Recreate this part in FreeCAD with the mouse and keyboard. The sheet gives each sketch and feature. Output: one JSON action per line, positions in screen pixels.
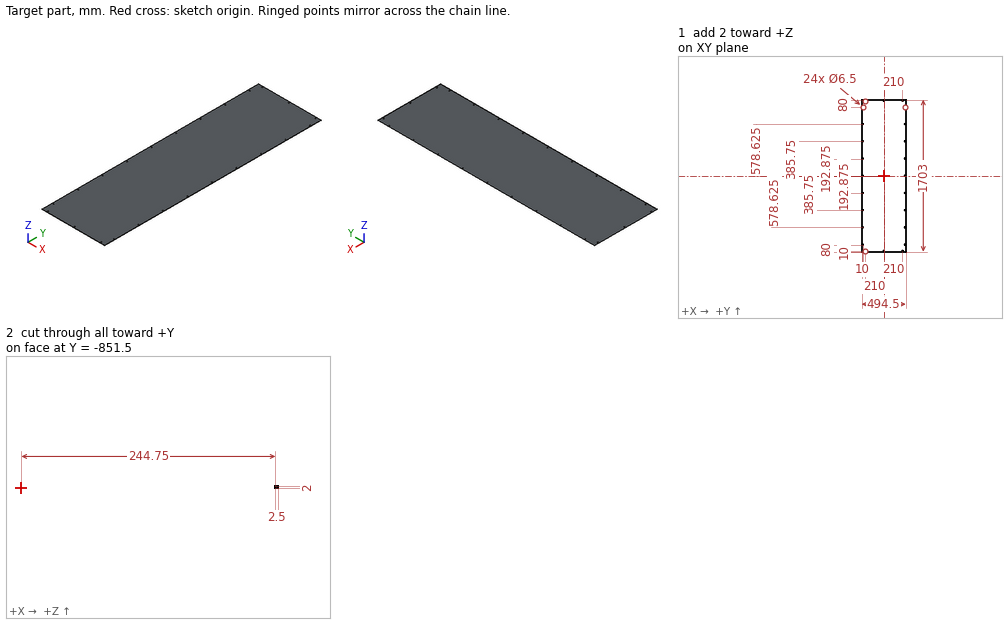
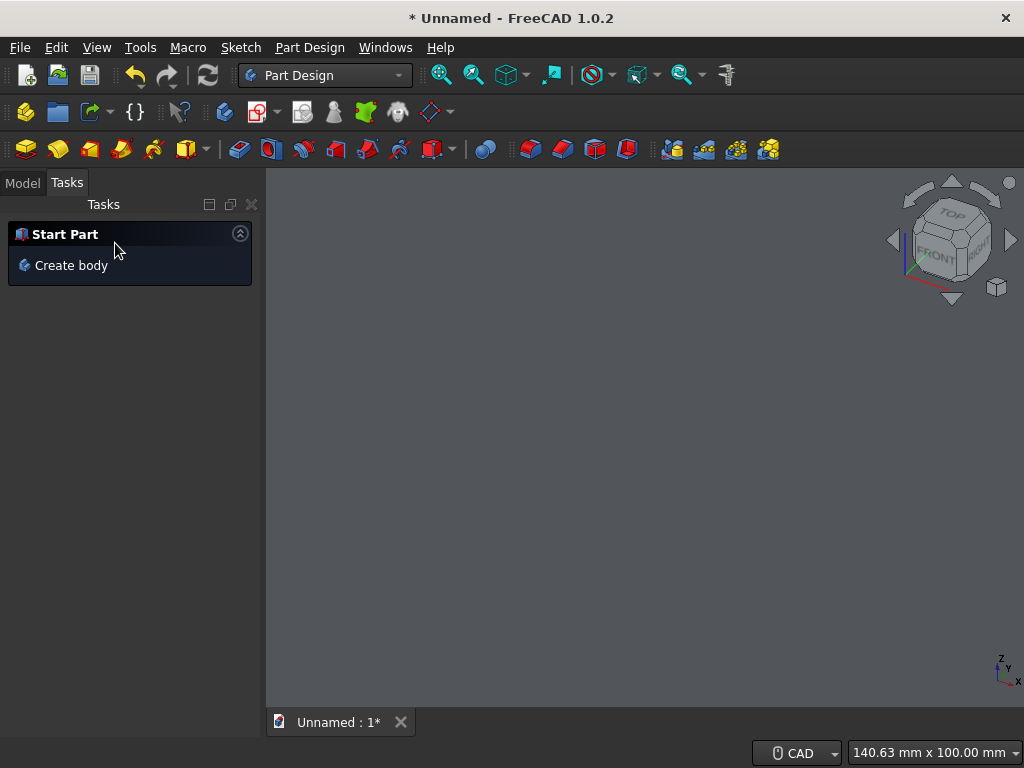
{"action": "left_click", "coordinate": [442, 76]}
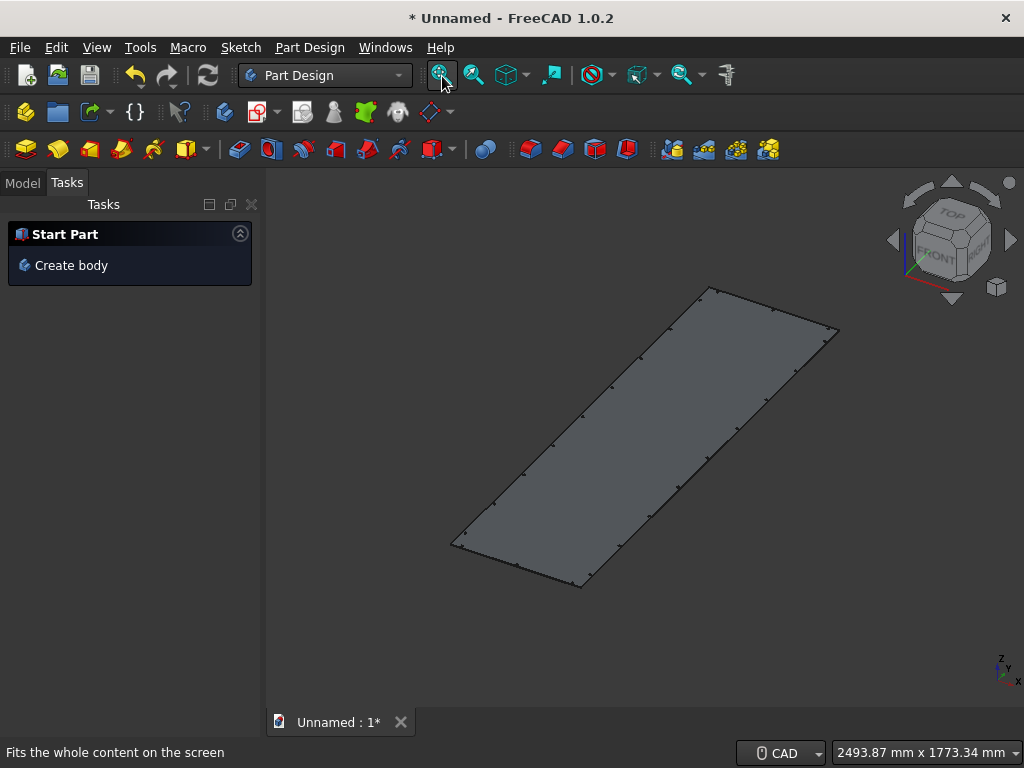
{"action": "scroll", "coordinate": [571, 584], "scroll_direction": "up", "scroll_amount": 15}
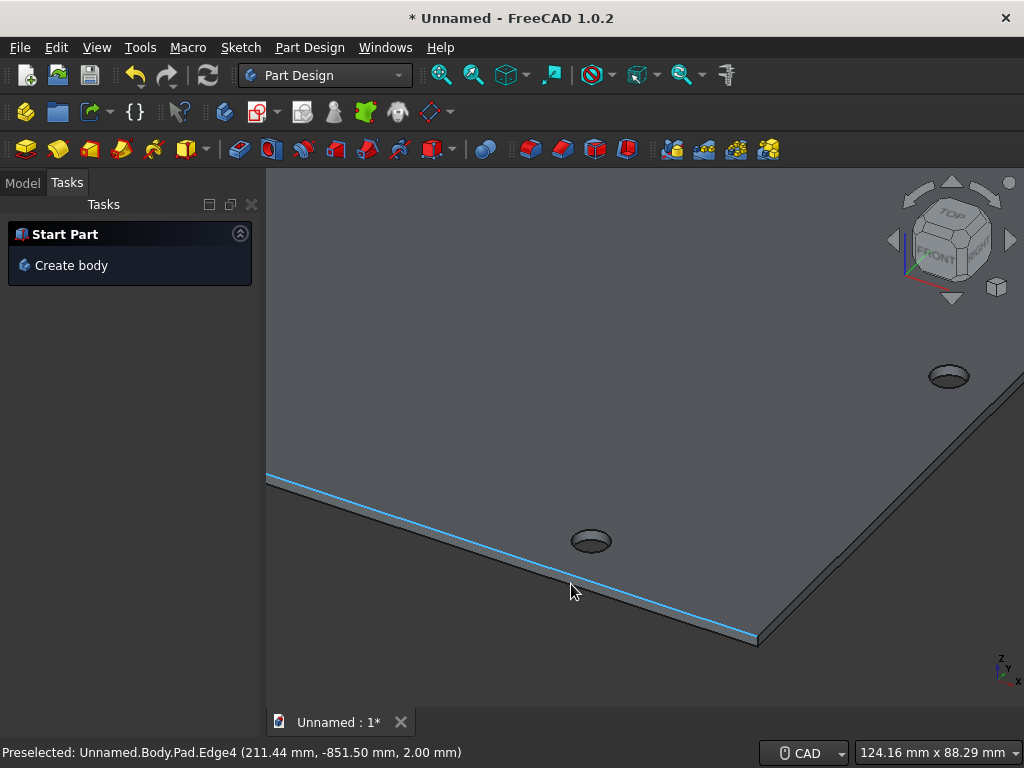
{"action": "scroll", "coordinate": [571, 579], "scroll_direction": "up", "scroll_amount": 4}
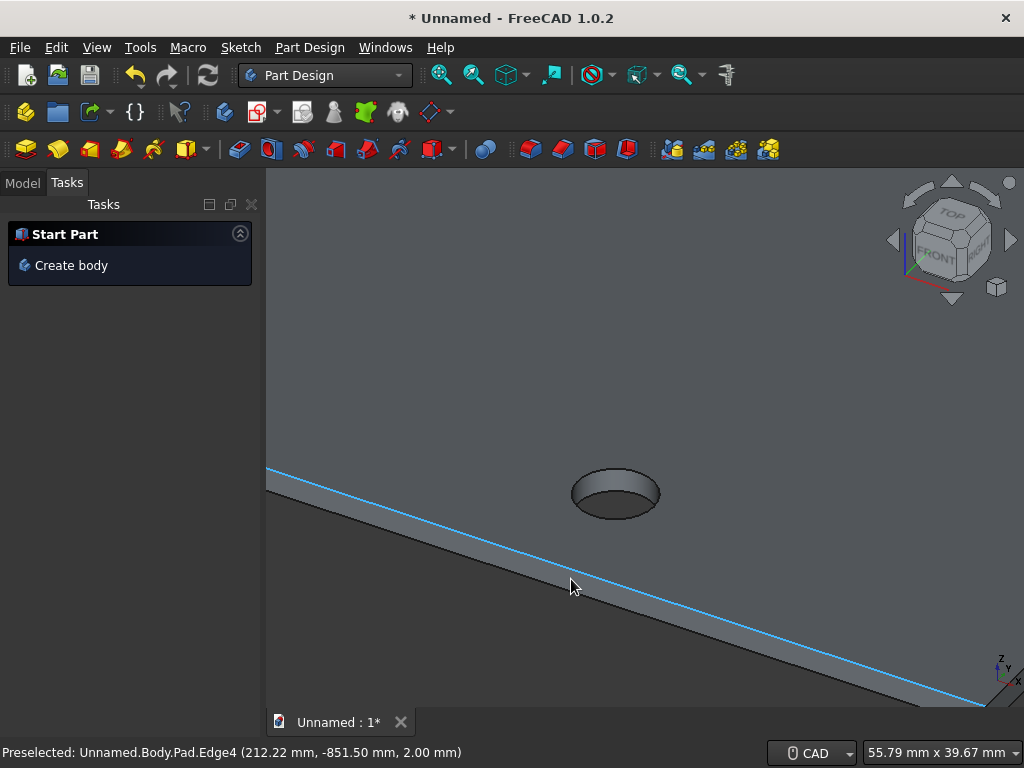
{"action": "left_click", "coordinate": [570, 579]}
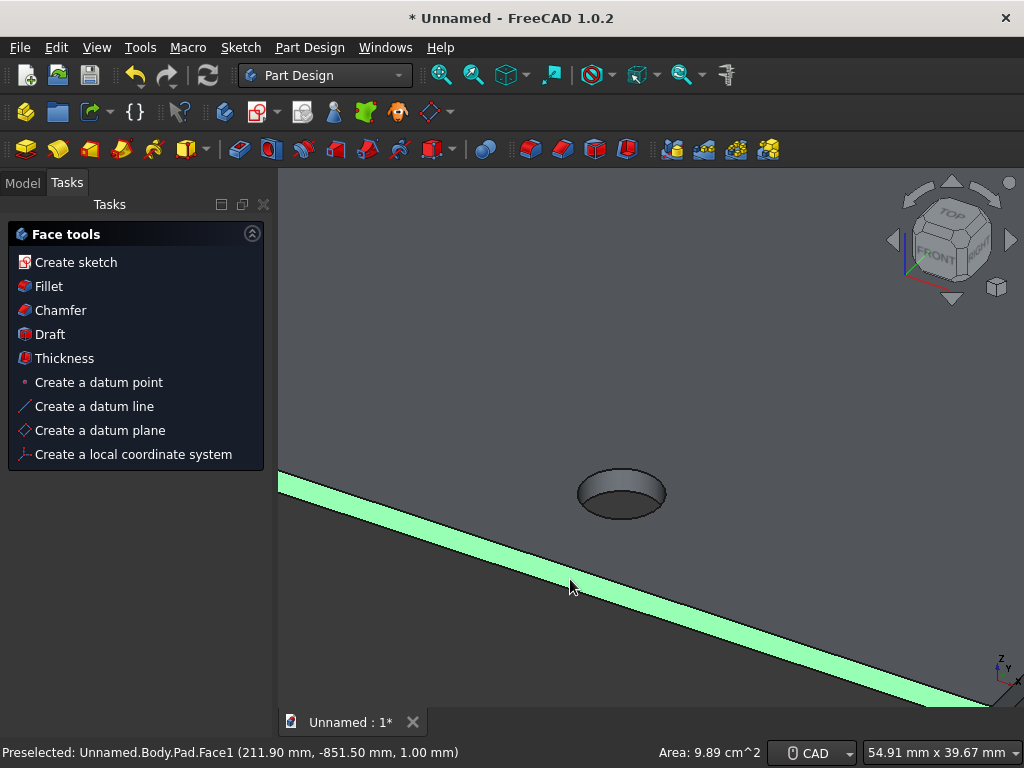
{"action": "left_click", "coordinate": [258, 112]}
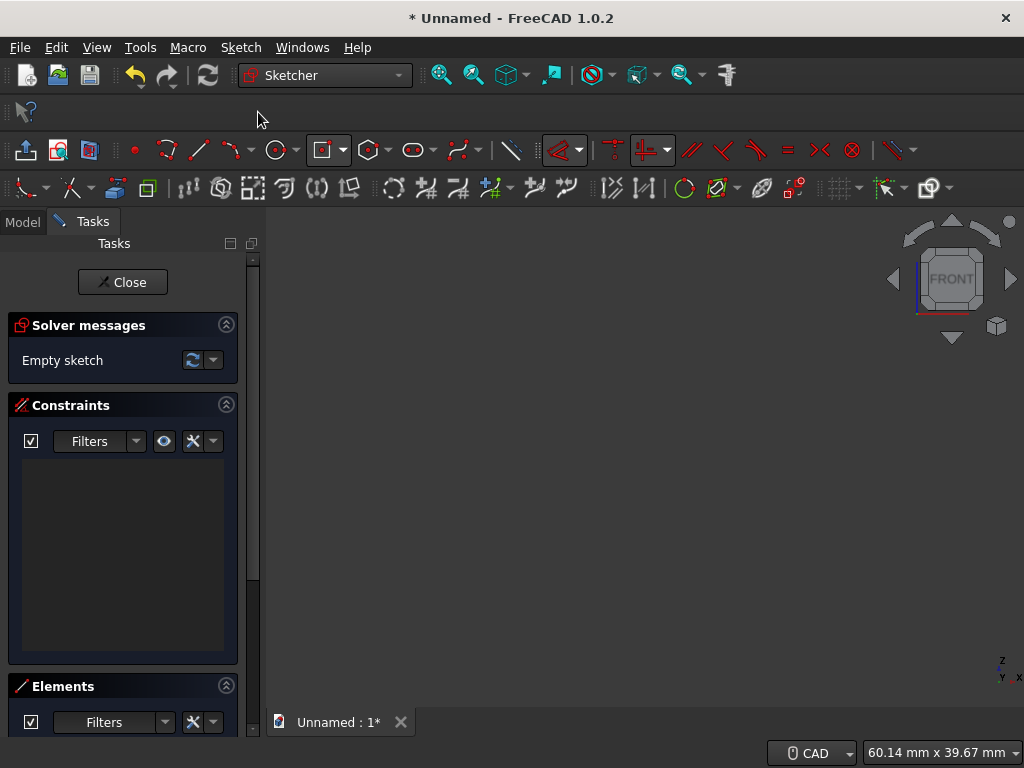
{"action": "scroll", "coordinate": [576, 457], "scroll_direction": "down", "scroll_amount": 5}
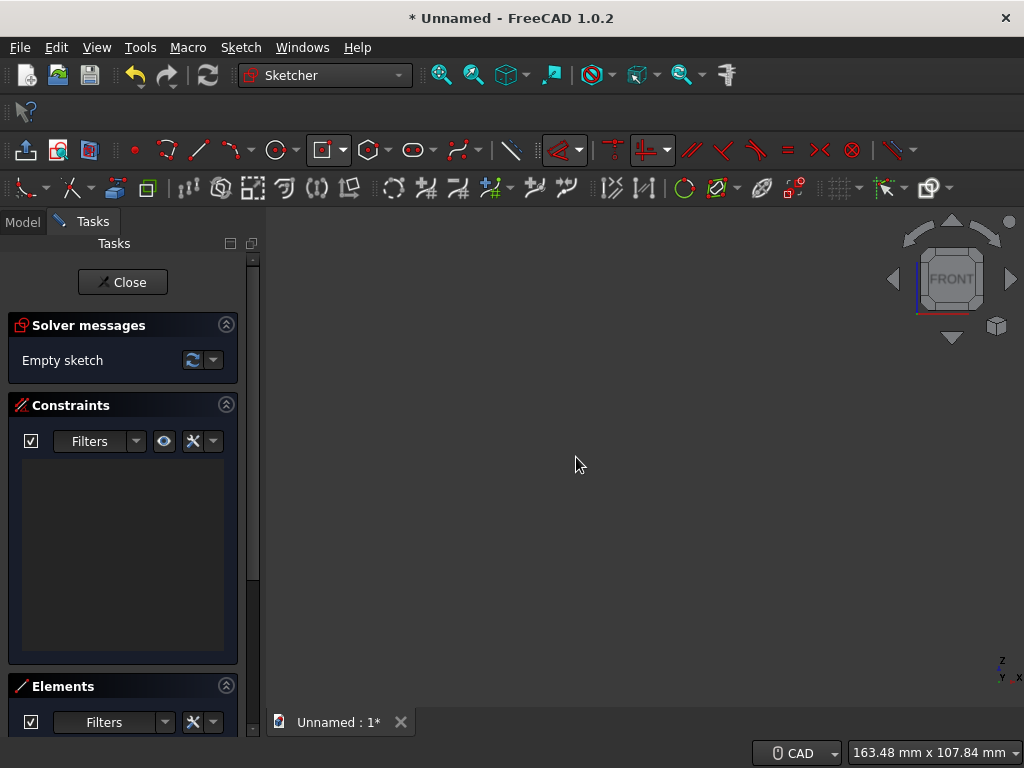
{"action": "scroll", "coordinate": [576, 457], "scroll_direction": "down", "scroll_amount": 5}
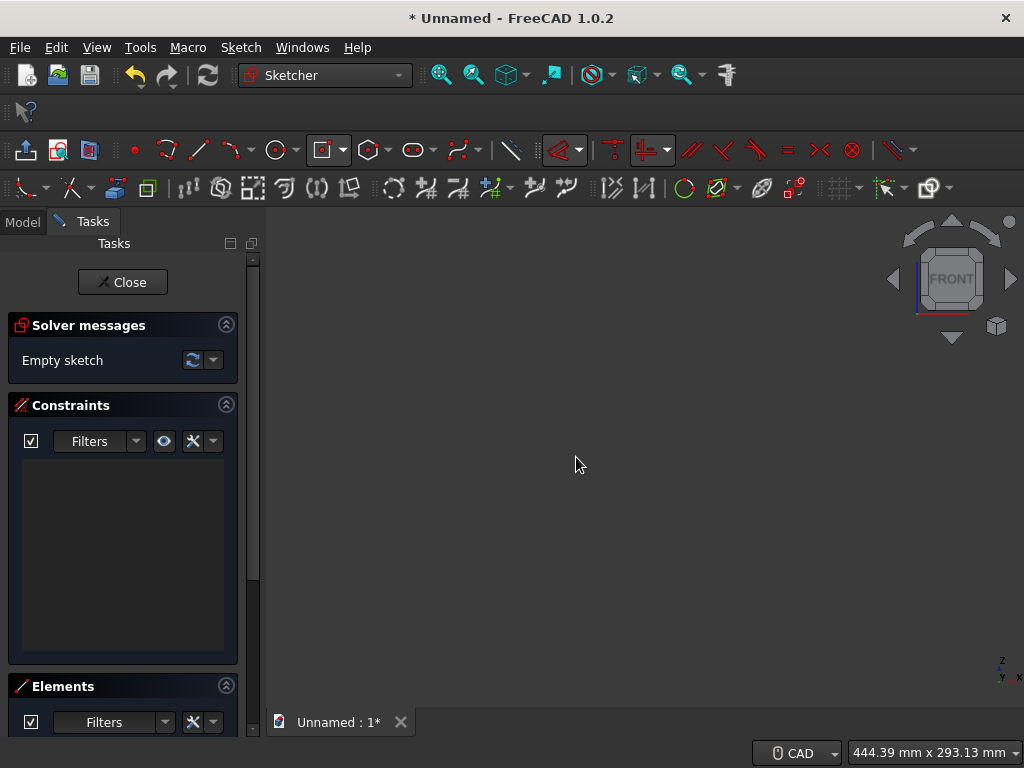
{"action": "scroll", "coordinate": [576, 457], "scroll_direction": "down", "scroll_amount": 5}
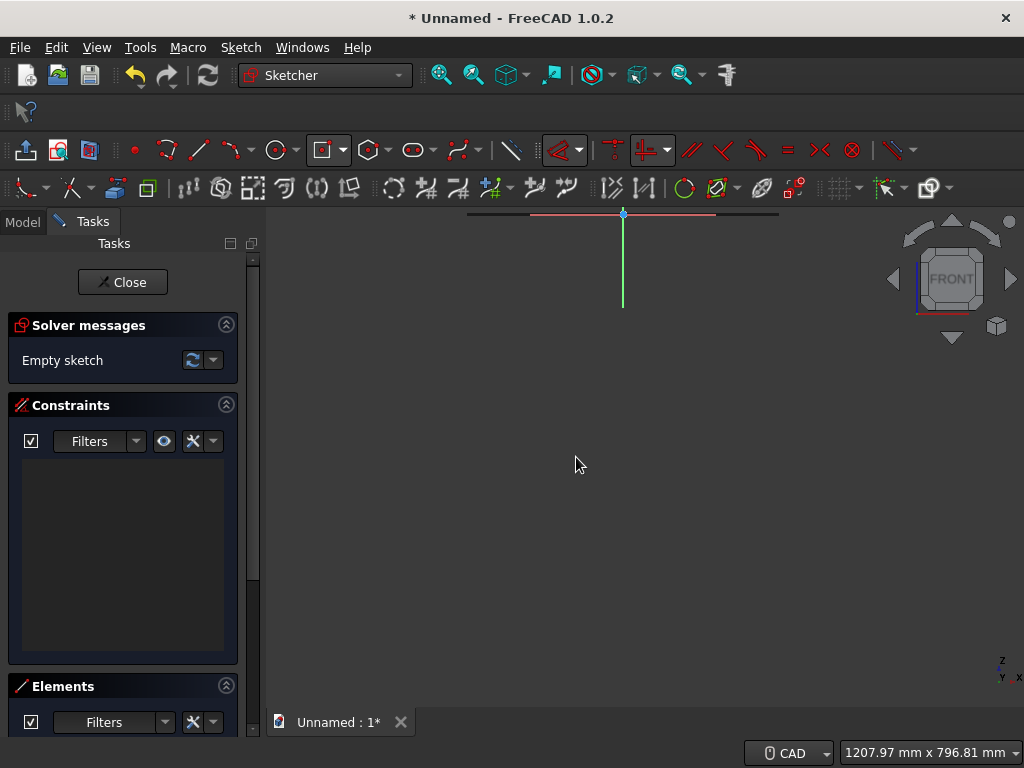
{"action": "scroll", "coordinate": [576, 457], "scroll_direction": "down", "scroll_amount": 5}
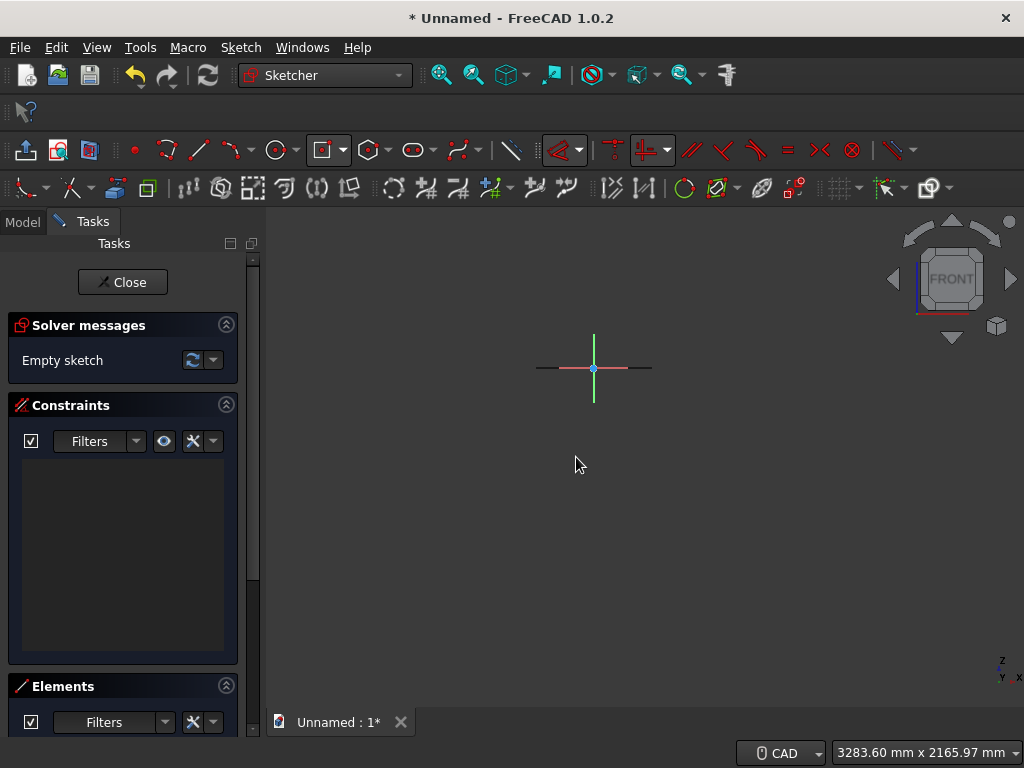
{"action": "scroll", "coordinate": [654, 363], "scroll_direction": "up", "scroll_amount": 15}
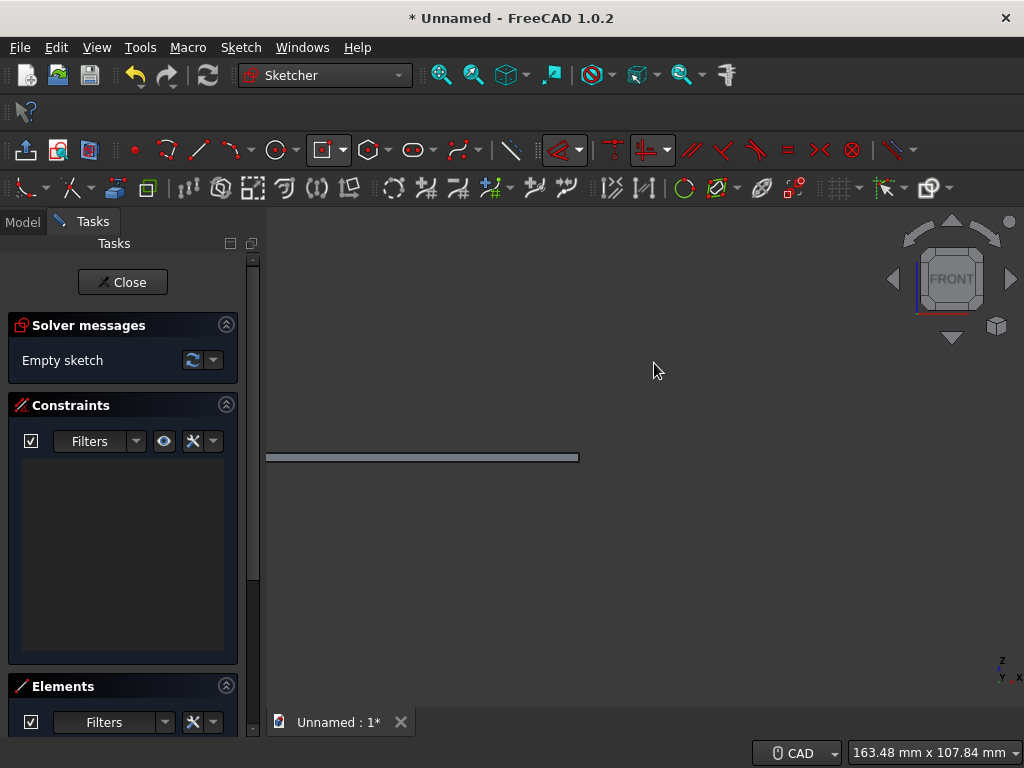
{"action": "left_click", "coordinate": [346, 150]}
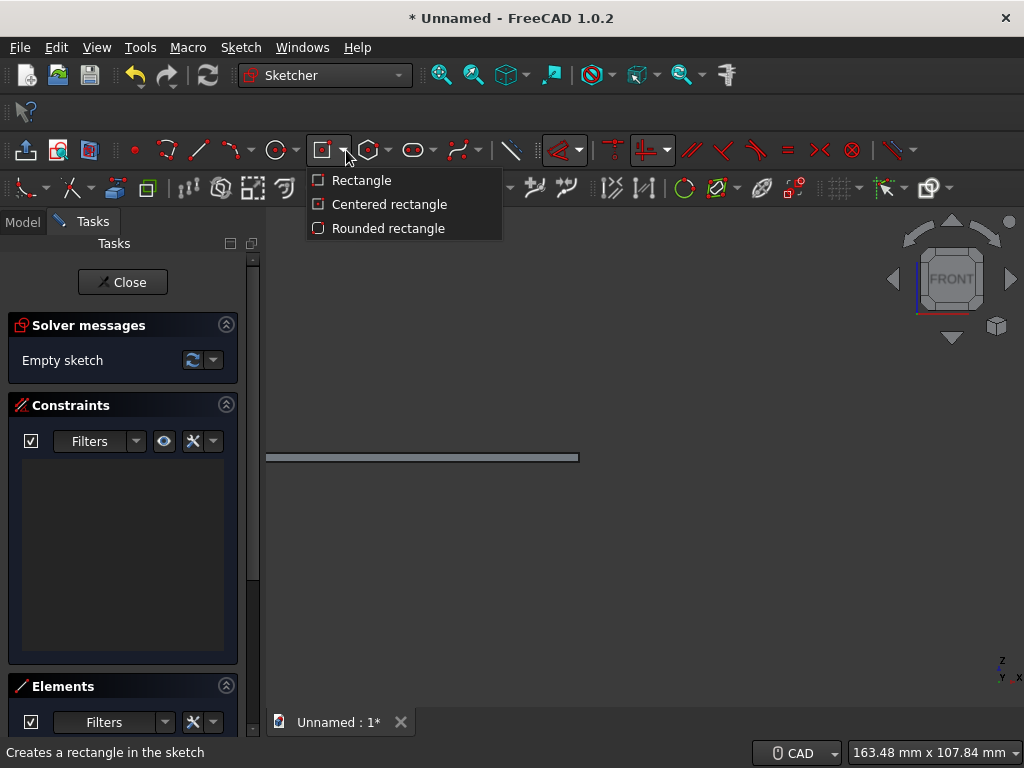
{"action": "left_click", "coordinate": [404, 180]}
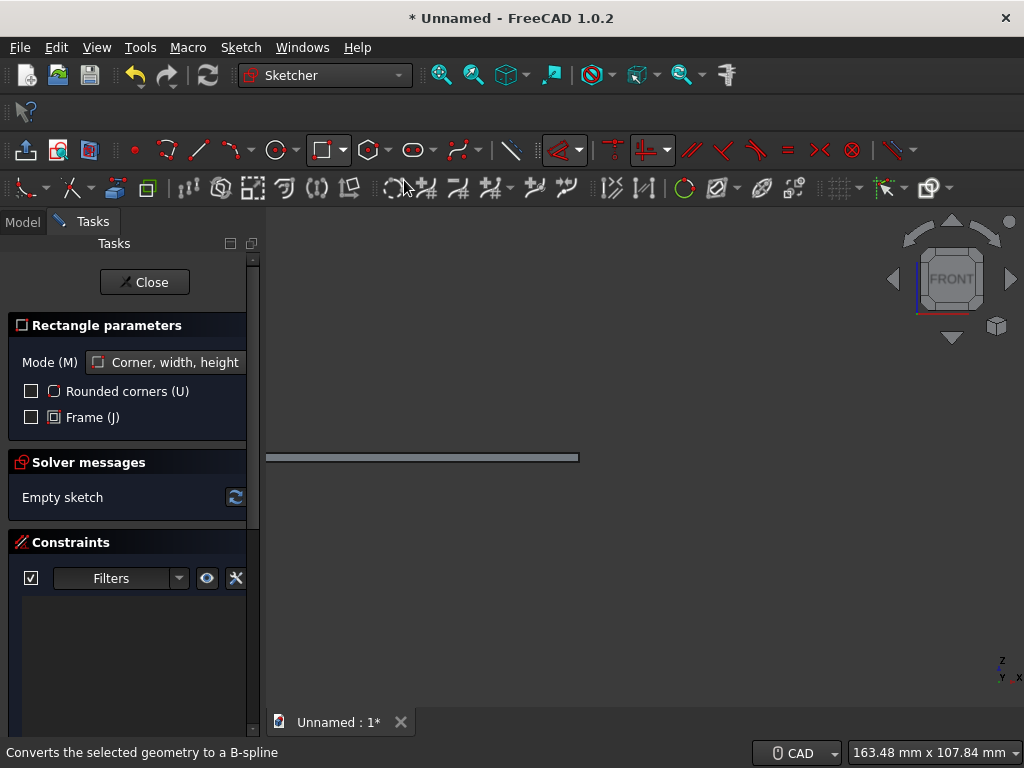
{"action": "scroll", "coordinate": [567, 453], "scroll_direction": "up", "scroll_amount": 3}